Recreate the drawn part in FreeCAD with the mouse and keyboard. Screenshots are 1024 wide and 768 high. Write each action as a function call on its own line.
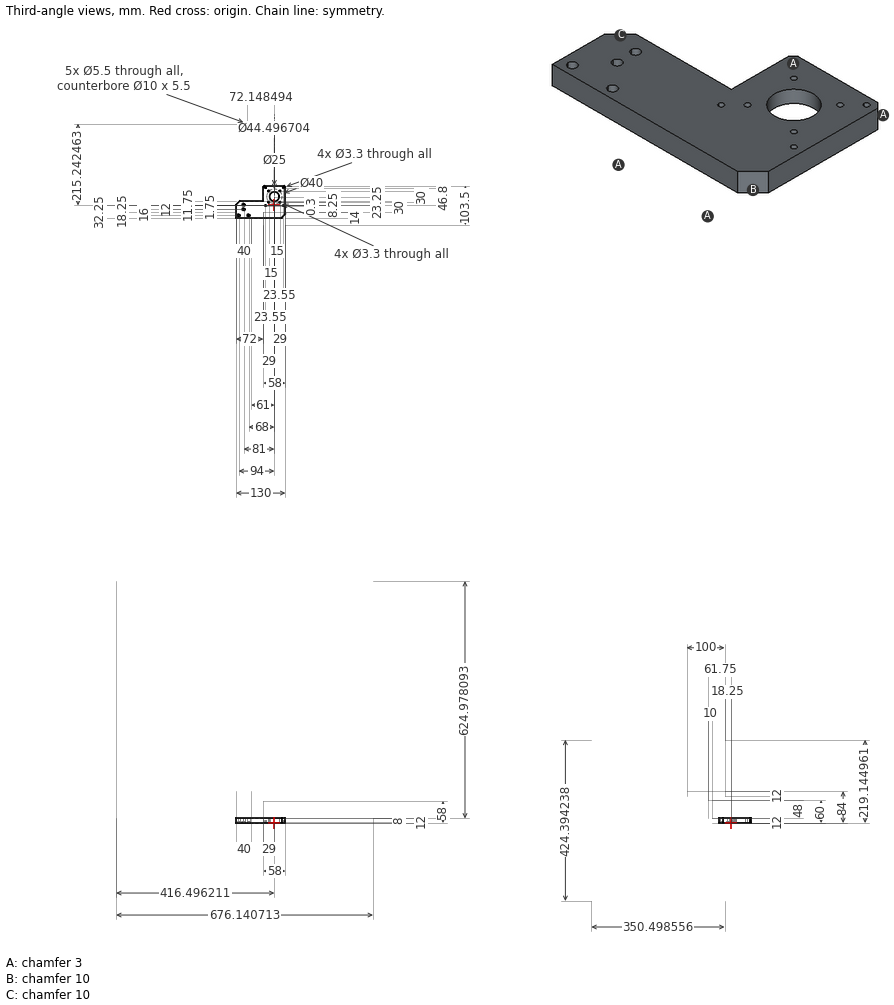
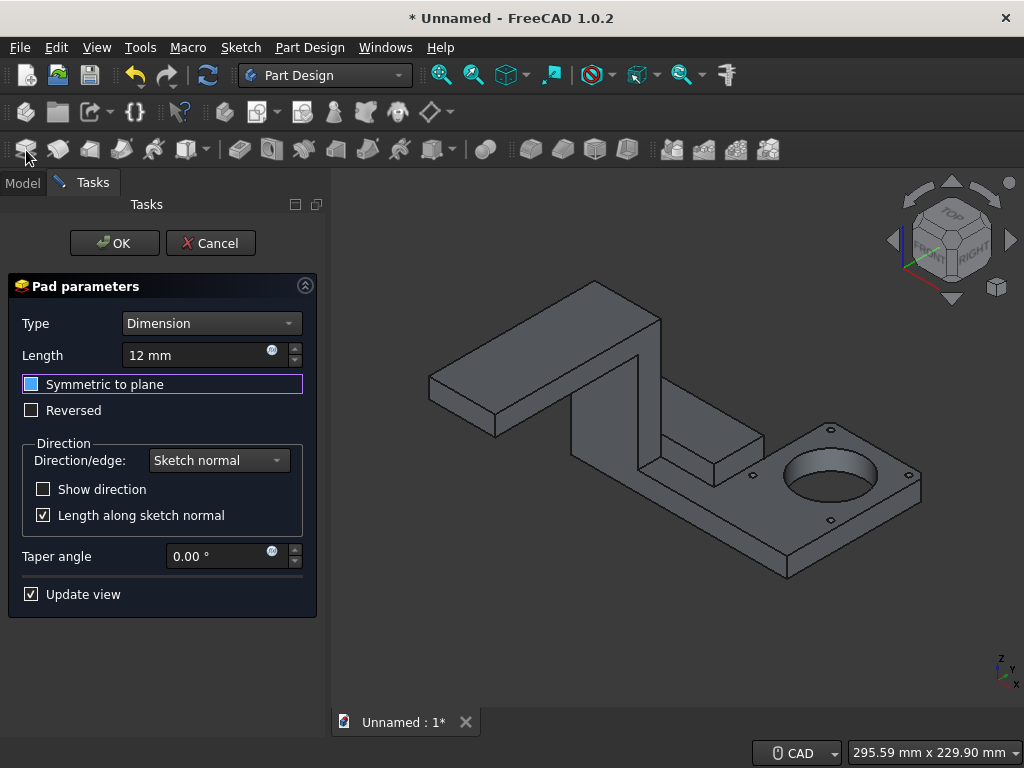
click(30, 410)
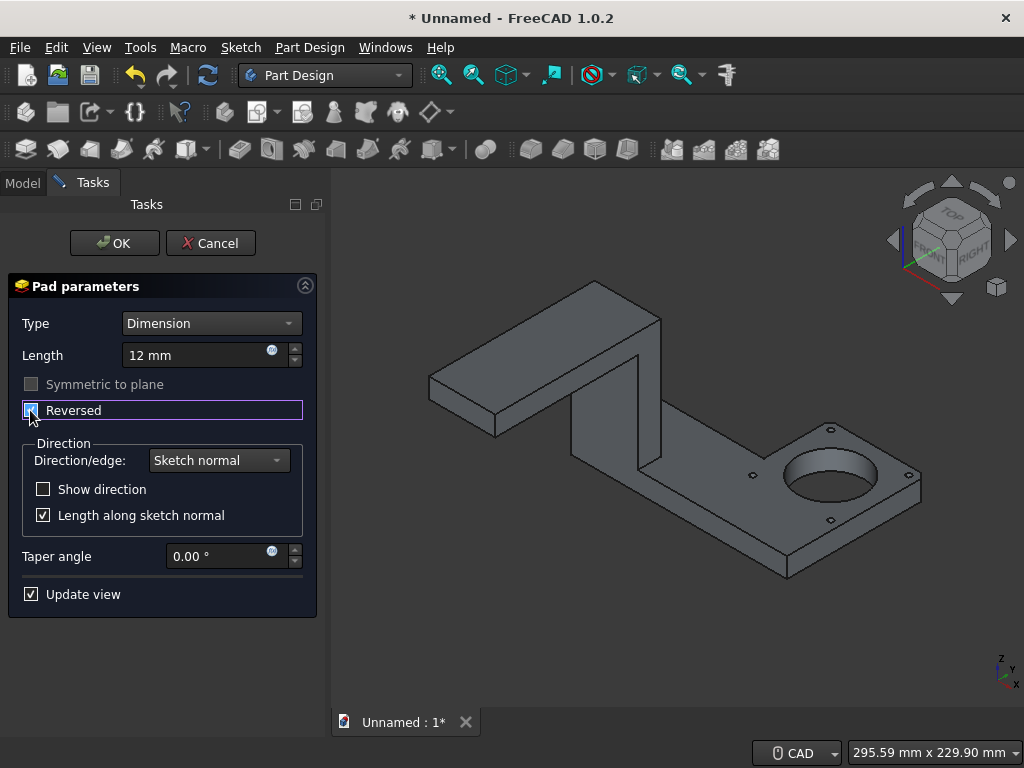
click(115, 243)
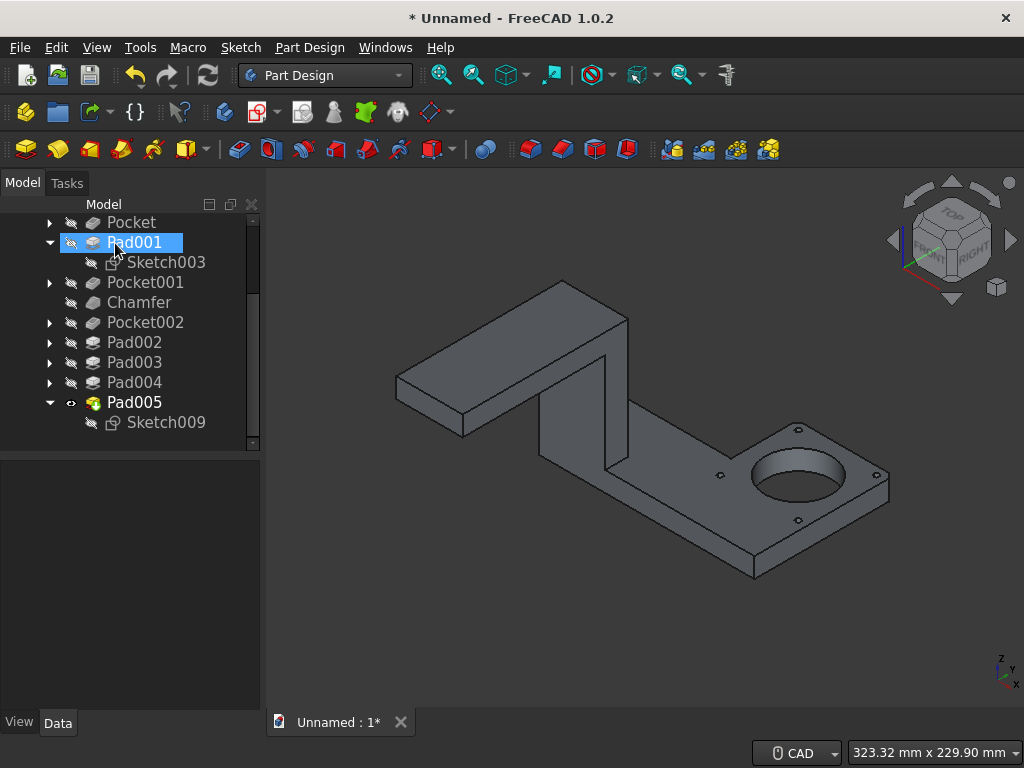
click(754, 567)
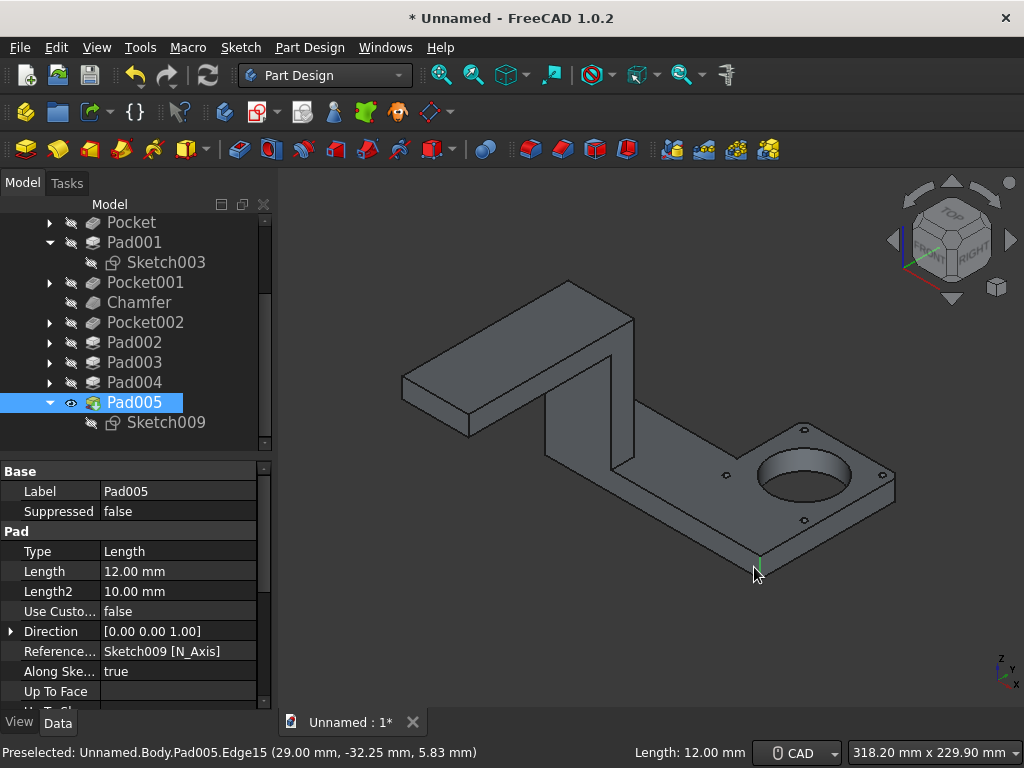
click(564, 150)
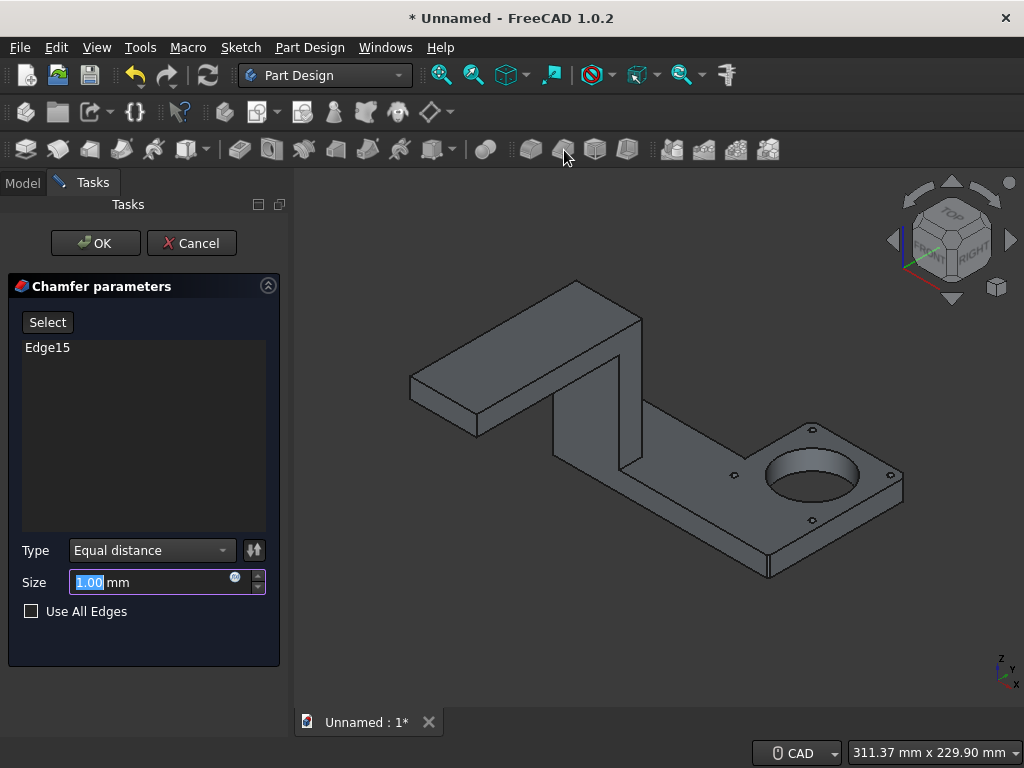
text(10)
key(Tab)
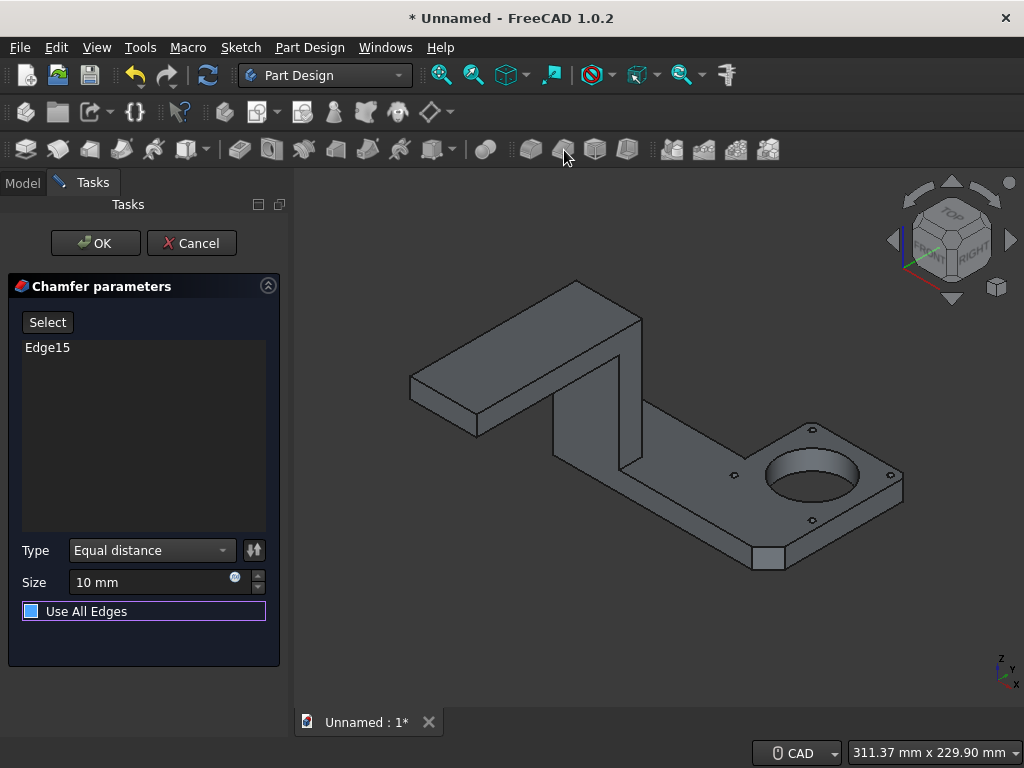
click(96, 243)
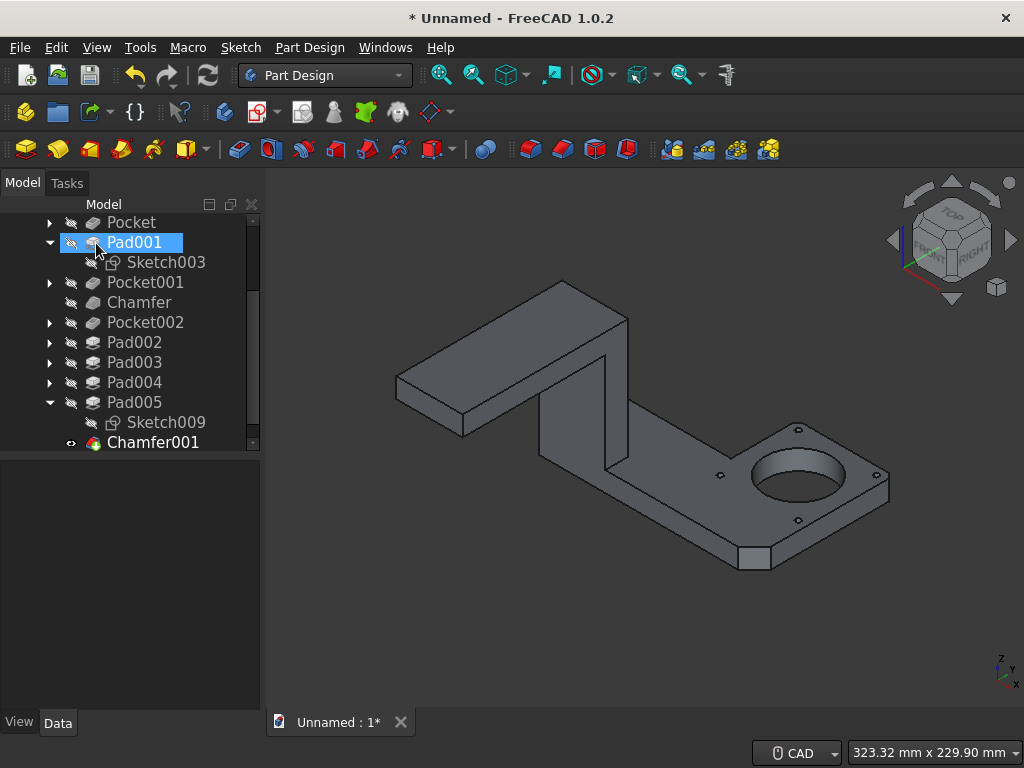
click(738, 511)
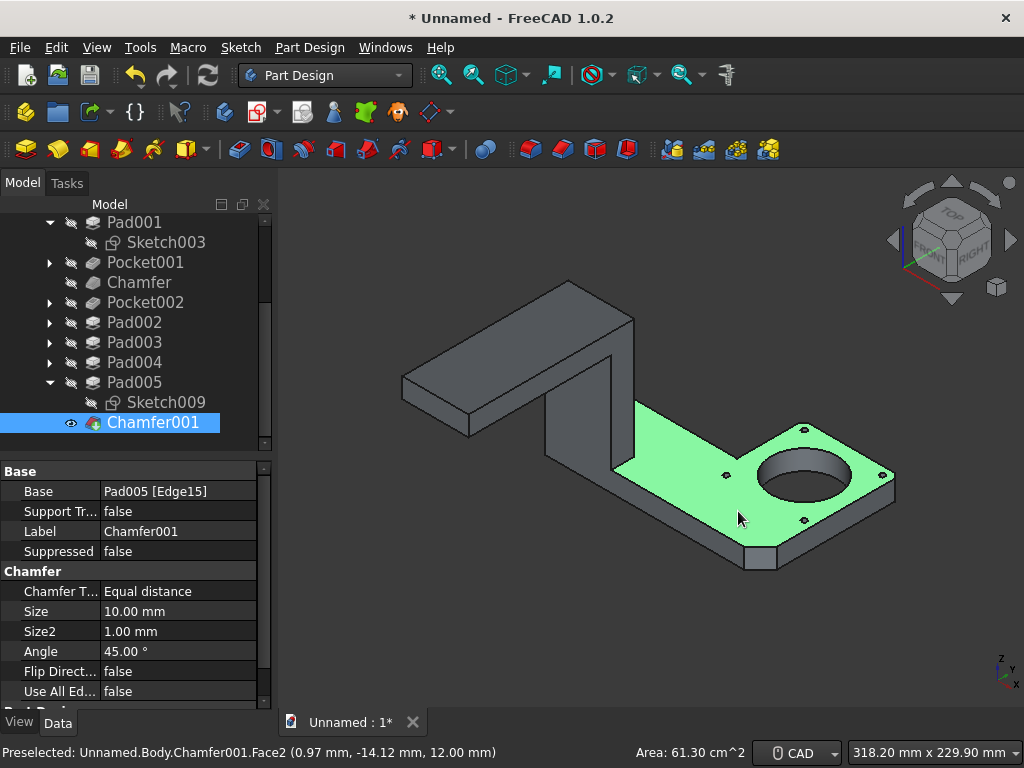
click(258, 112)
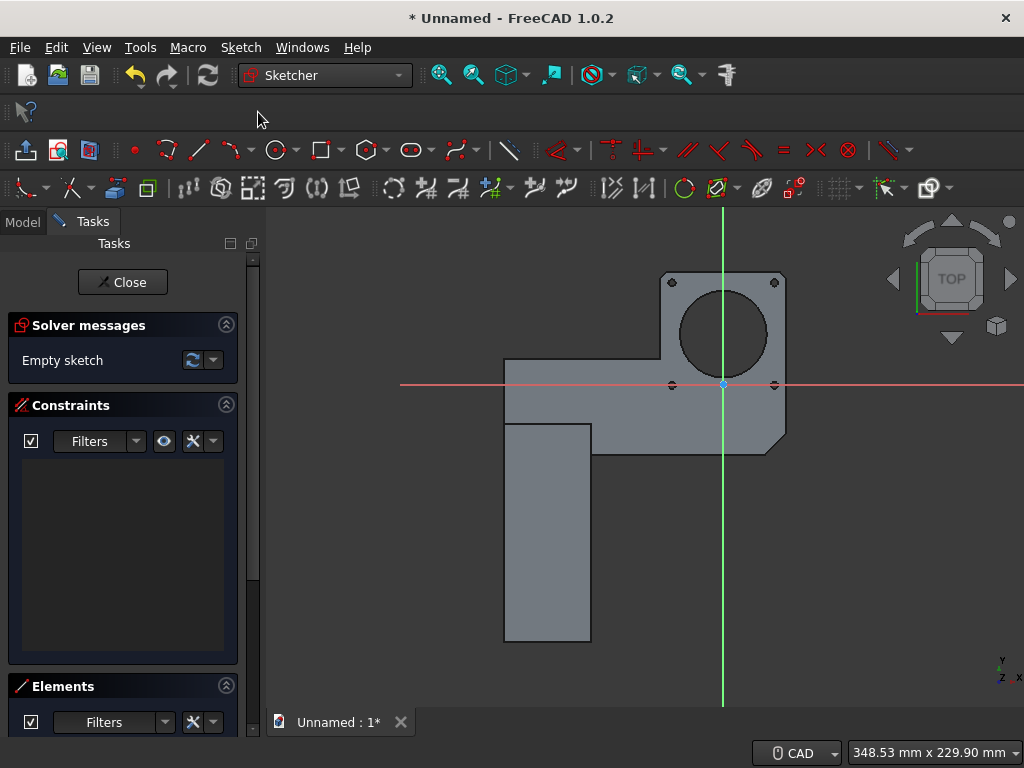
click(90, 150)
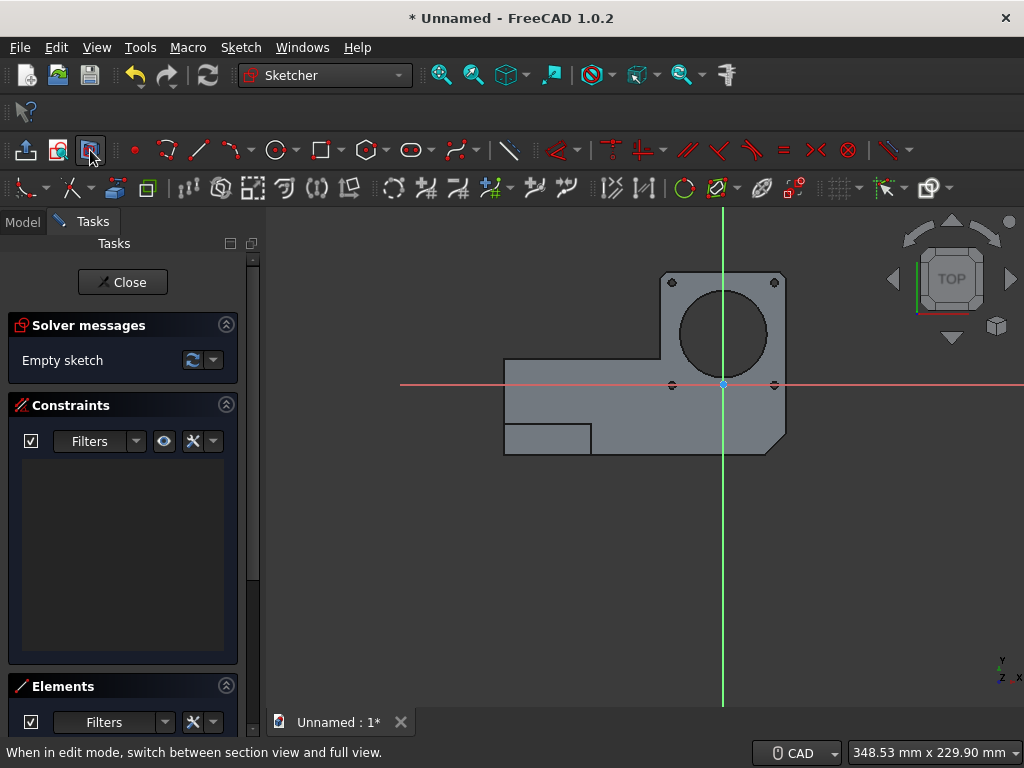
scroll(787, 283, up, 6)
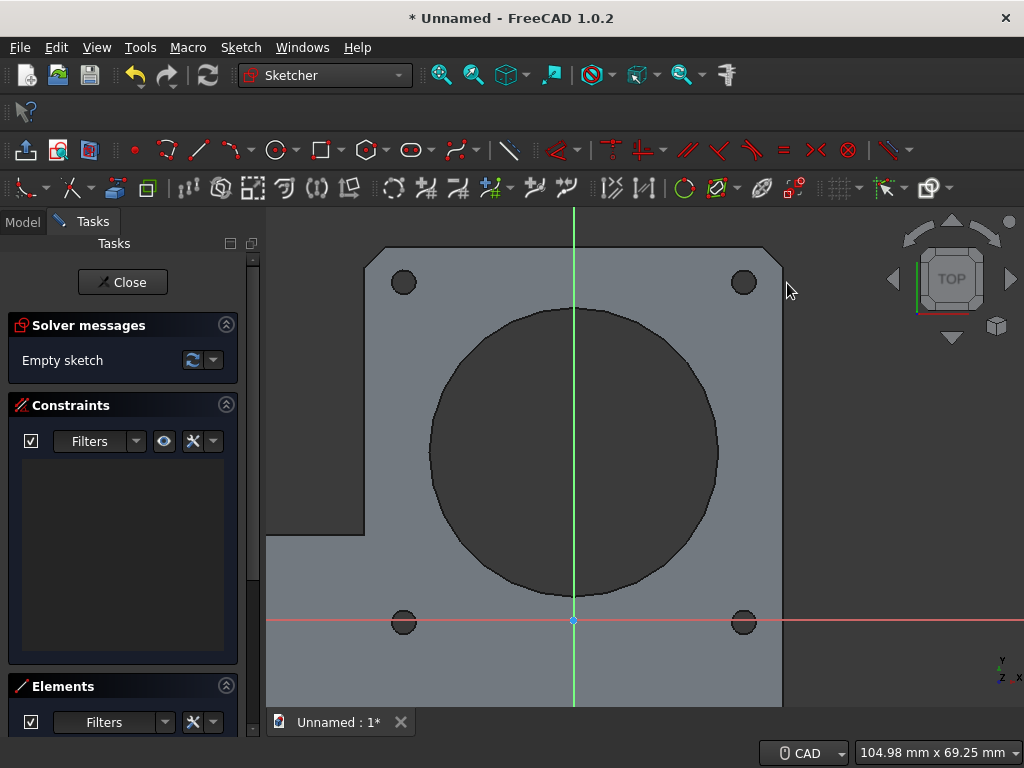
click(276, 150)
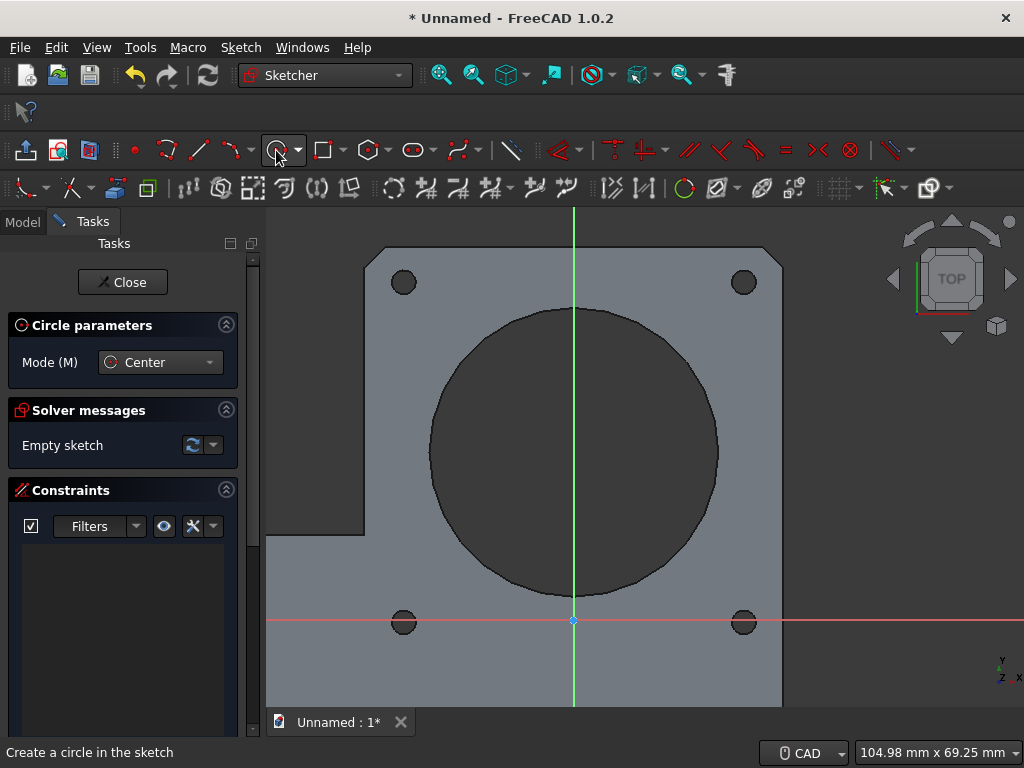
click(574, 452)
move(687, 339)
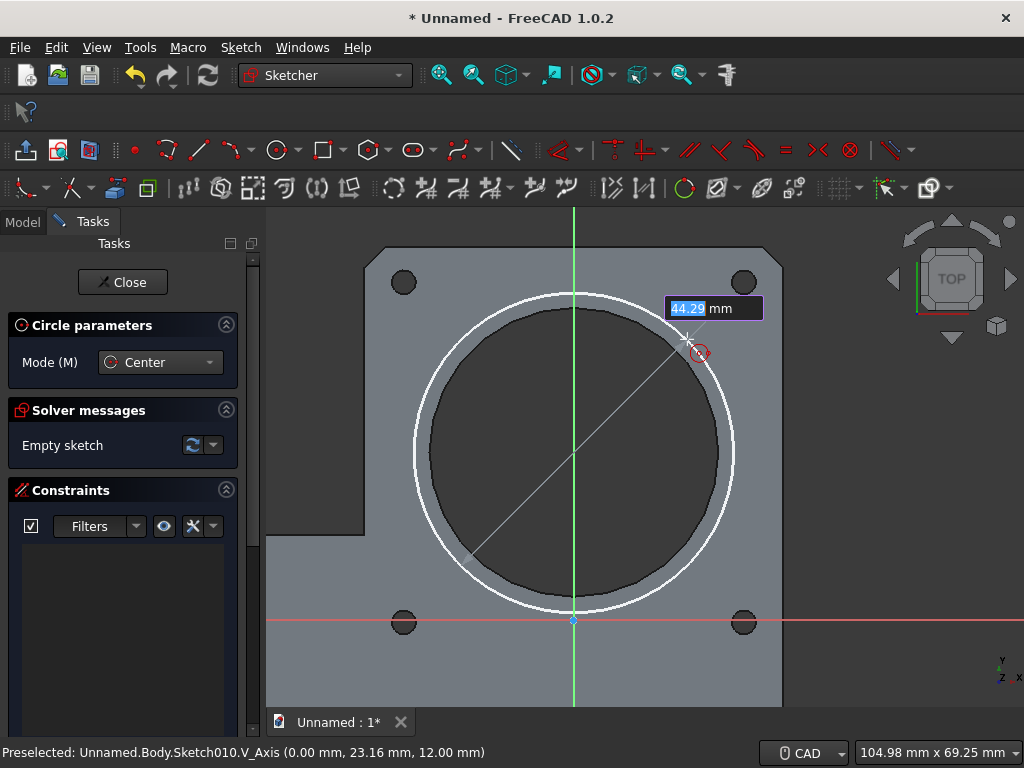
text(44.496704)
key(Return)